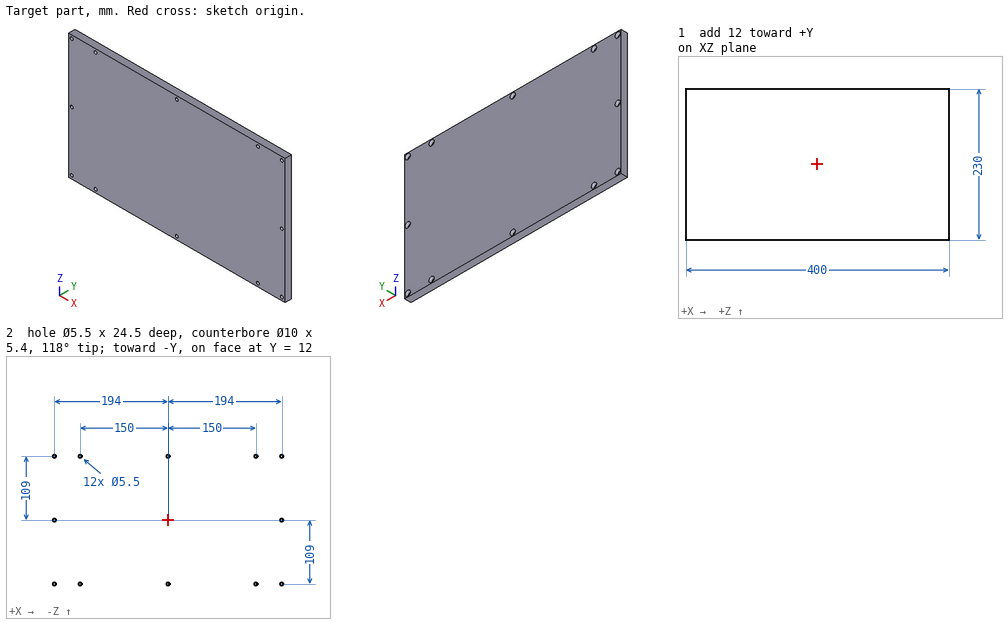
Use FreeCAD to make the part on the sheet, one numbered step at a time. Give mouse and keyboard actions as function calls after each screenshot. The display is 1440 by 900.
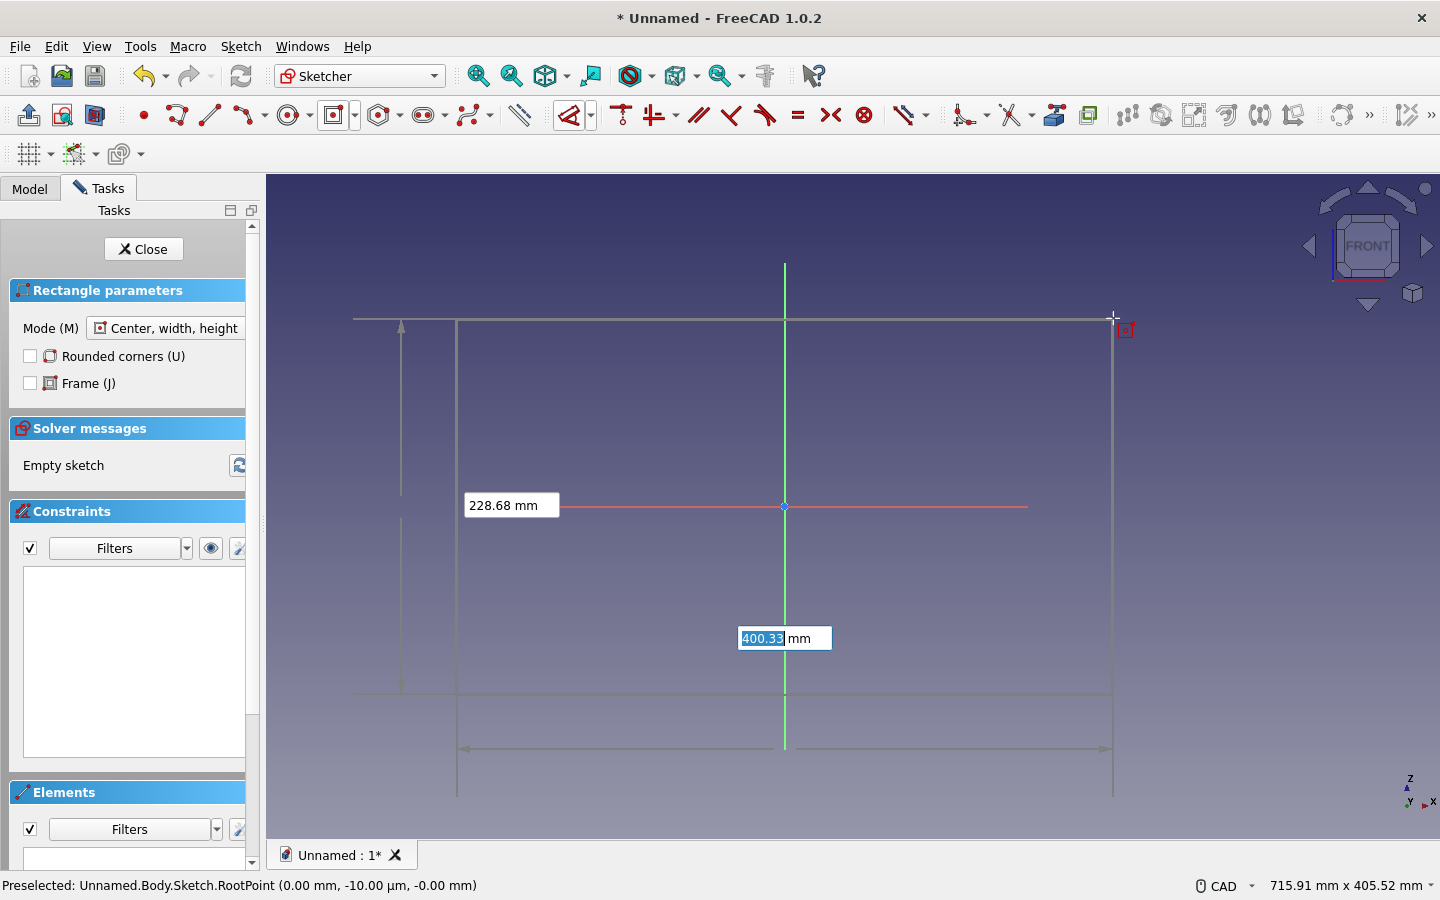
text(400)
key(Tab)
text(230)
key(Return)
key(Escape)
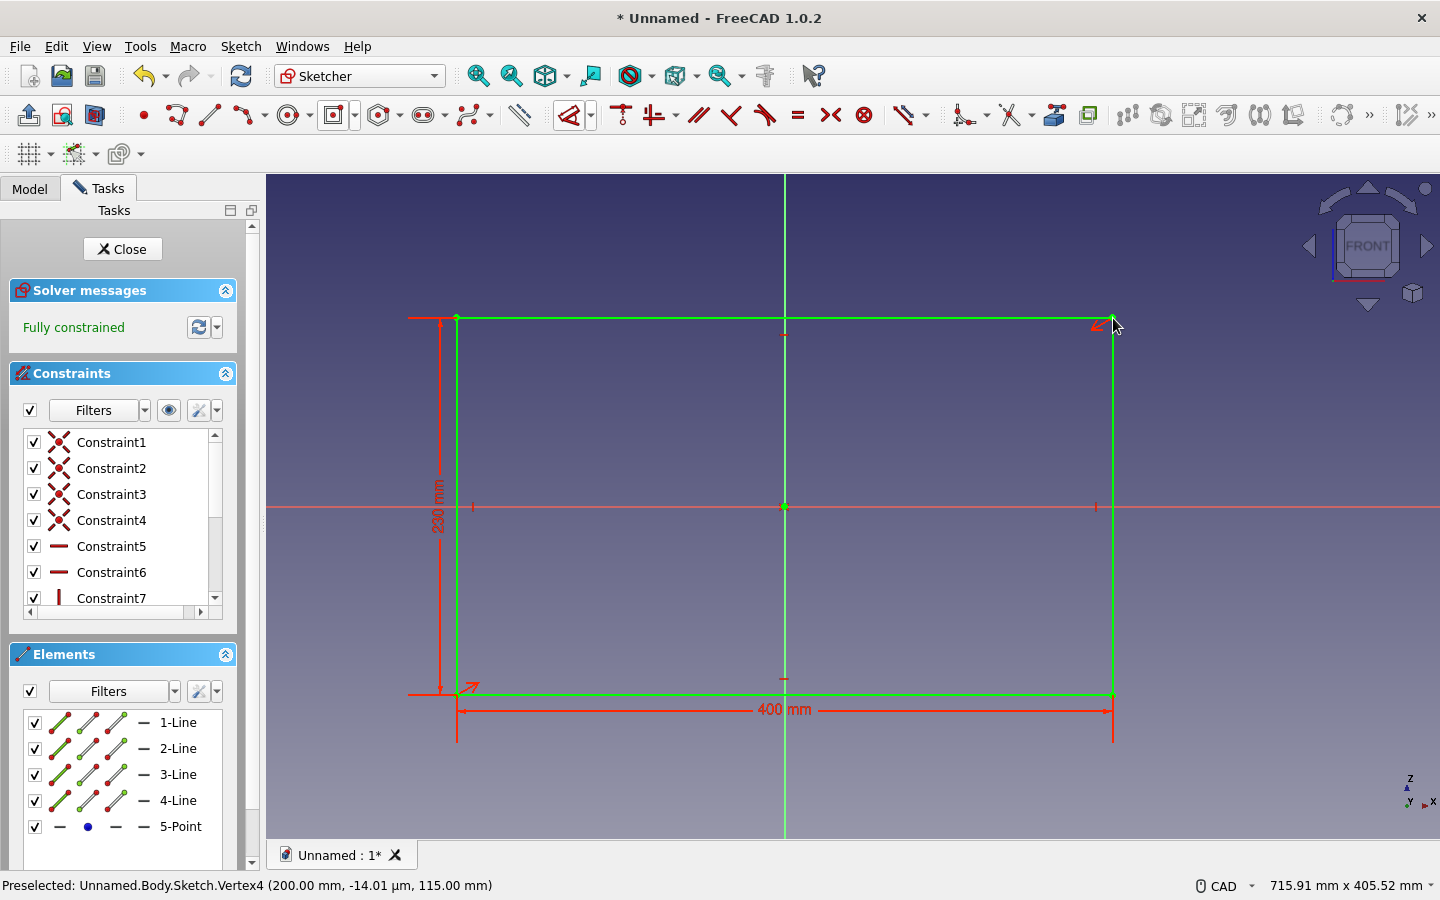
click(123, 249)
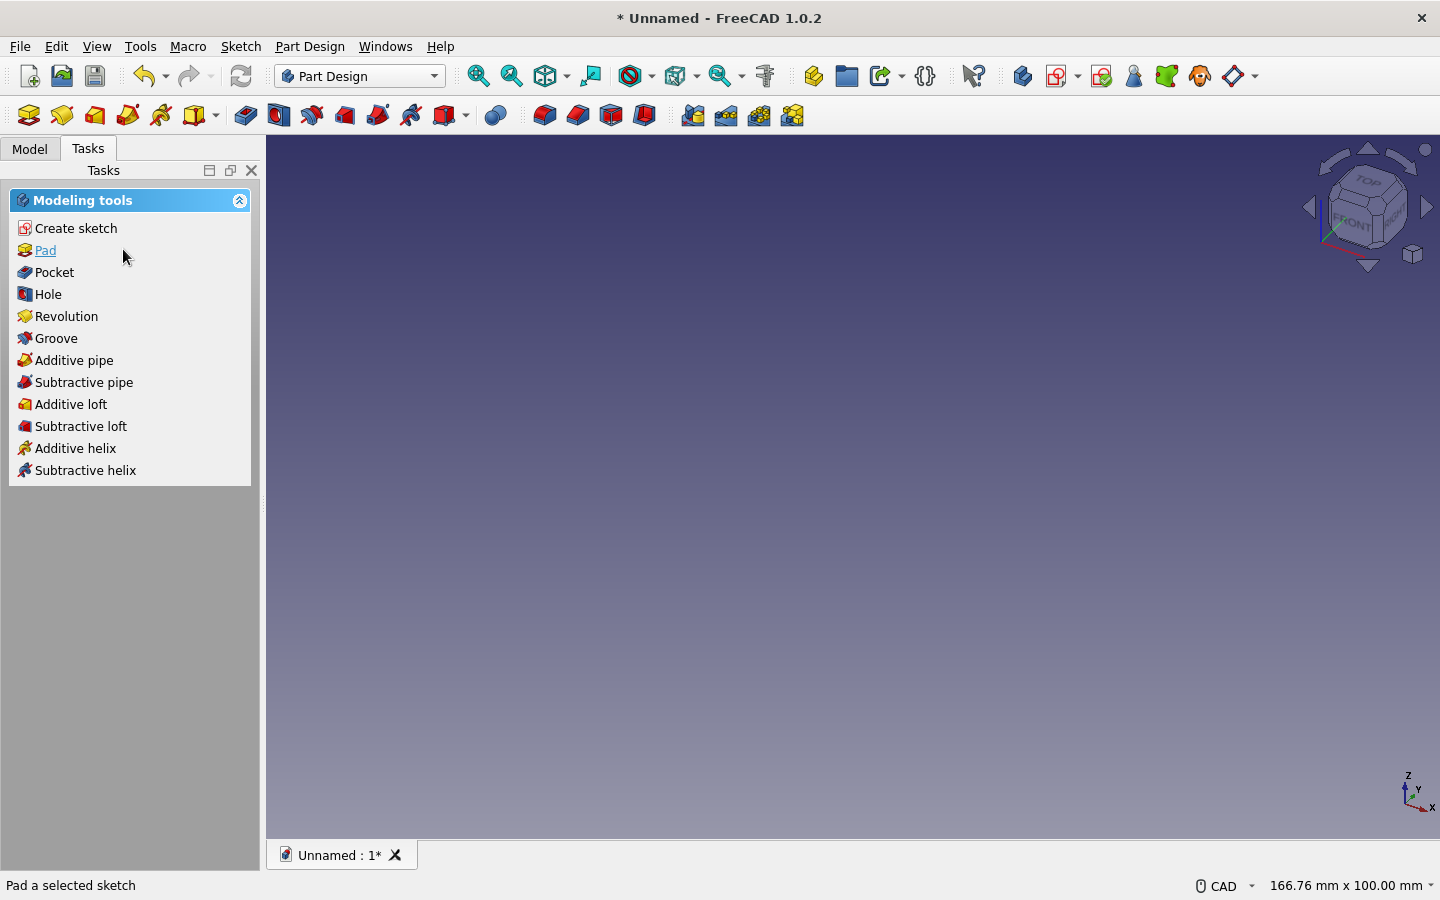
click(29, 116)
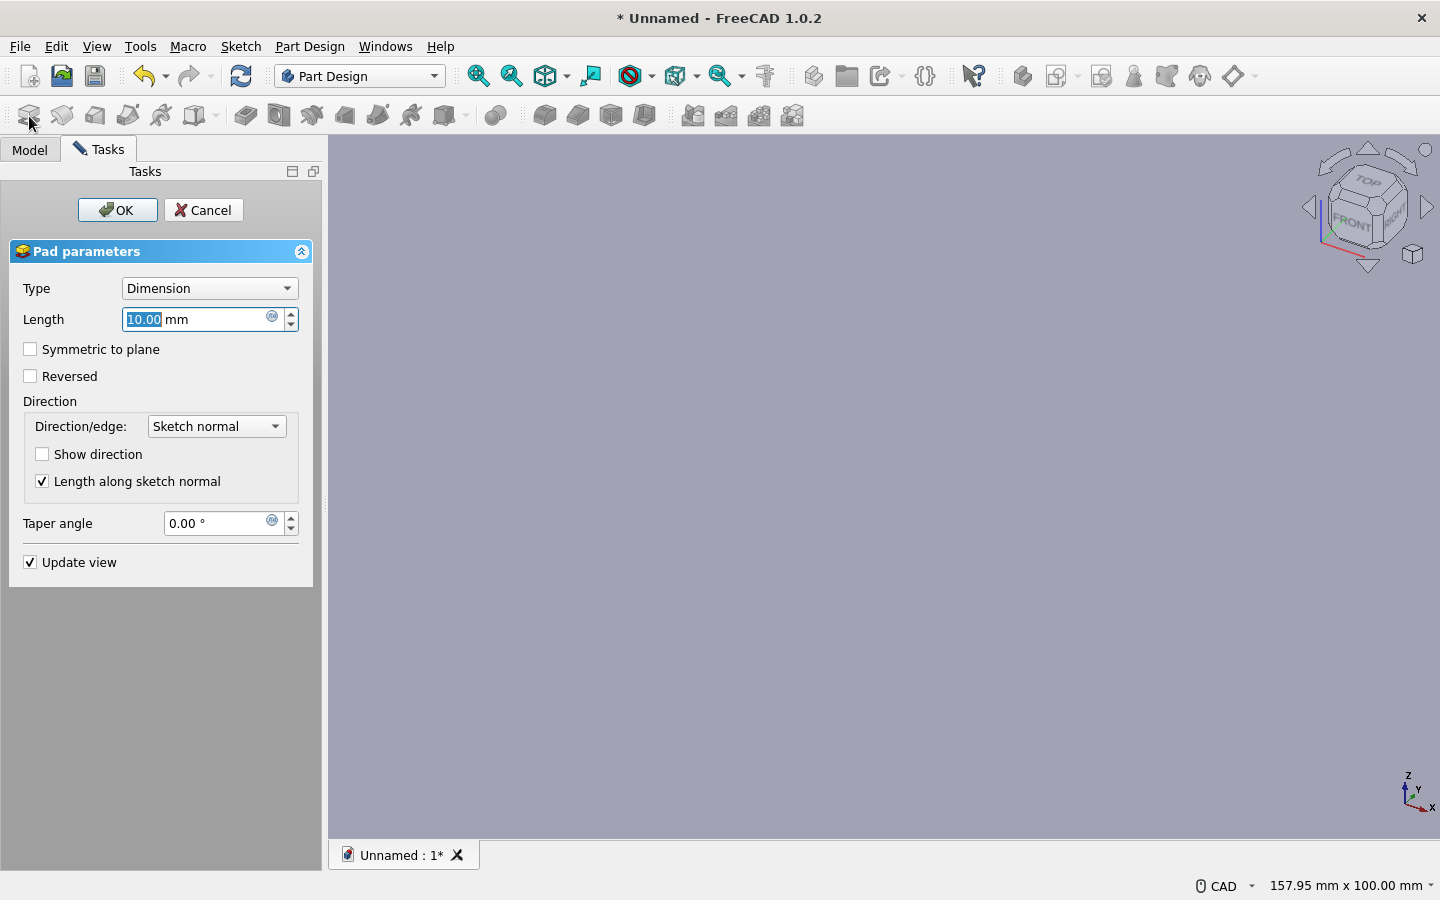
text(12)
key(Tab)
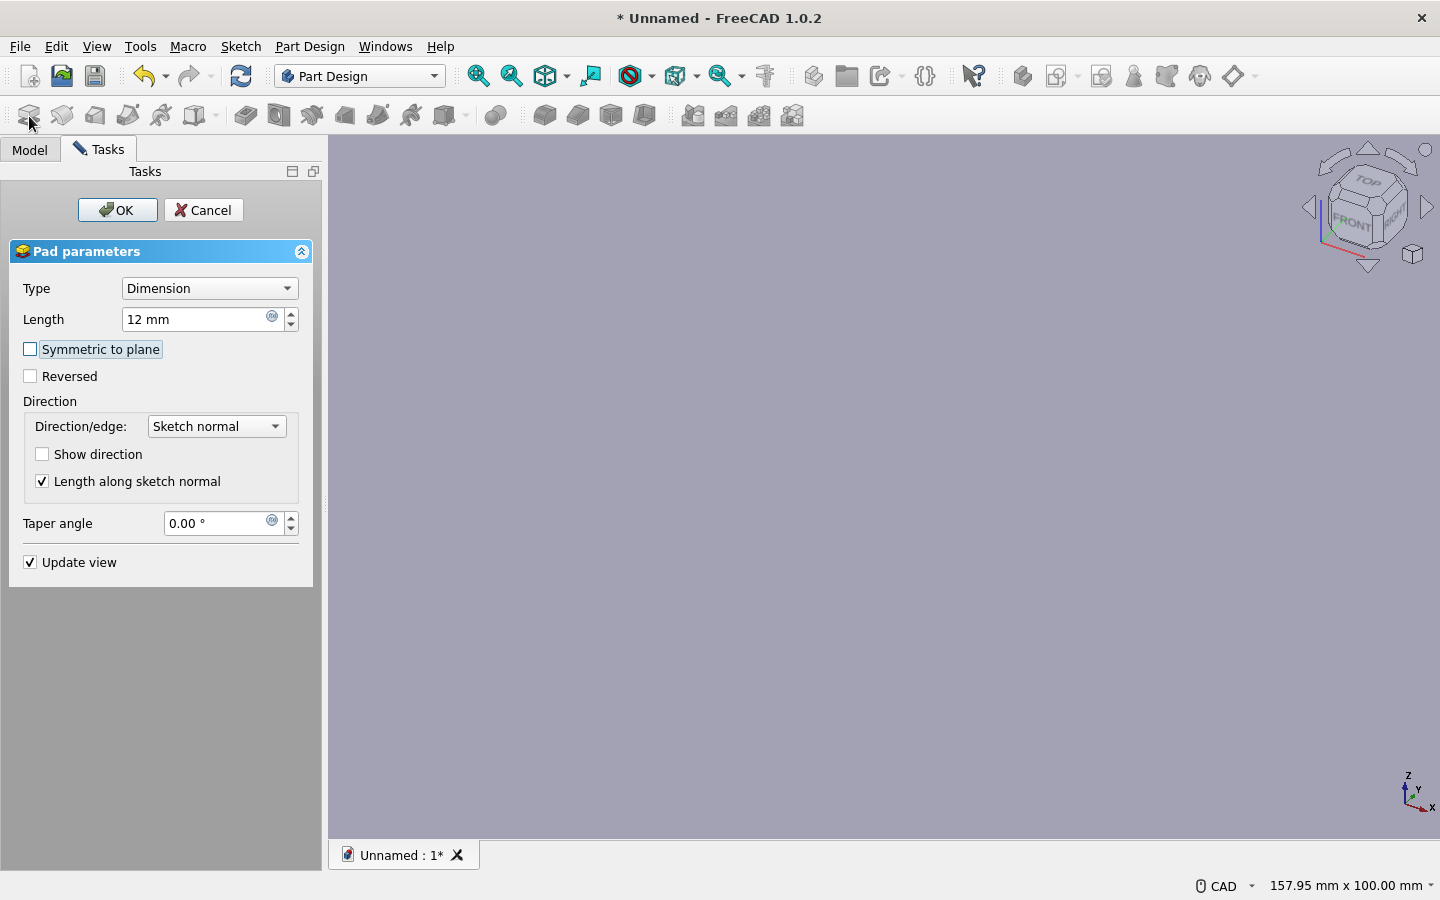
click(31, 376)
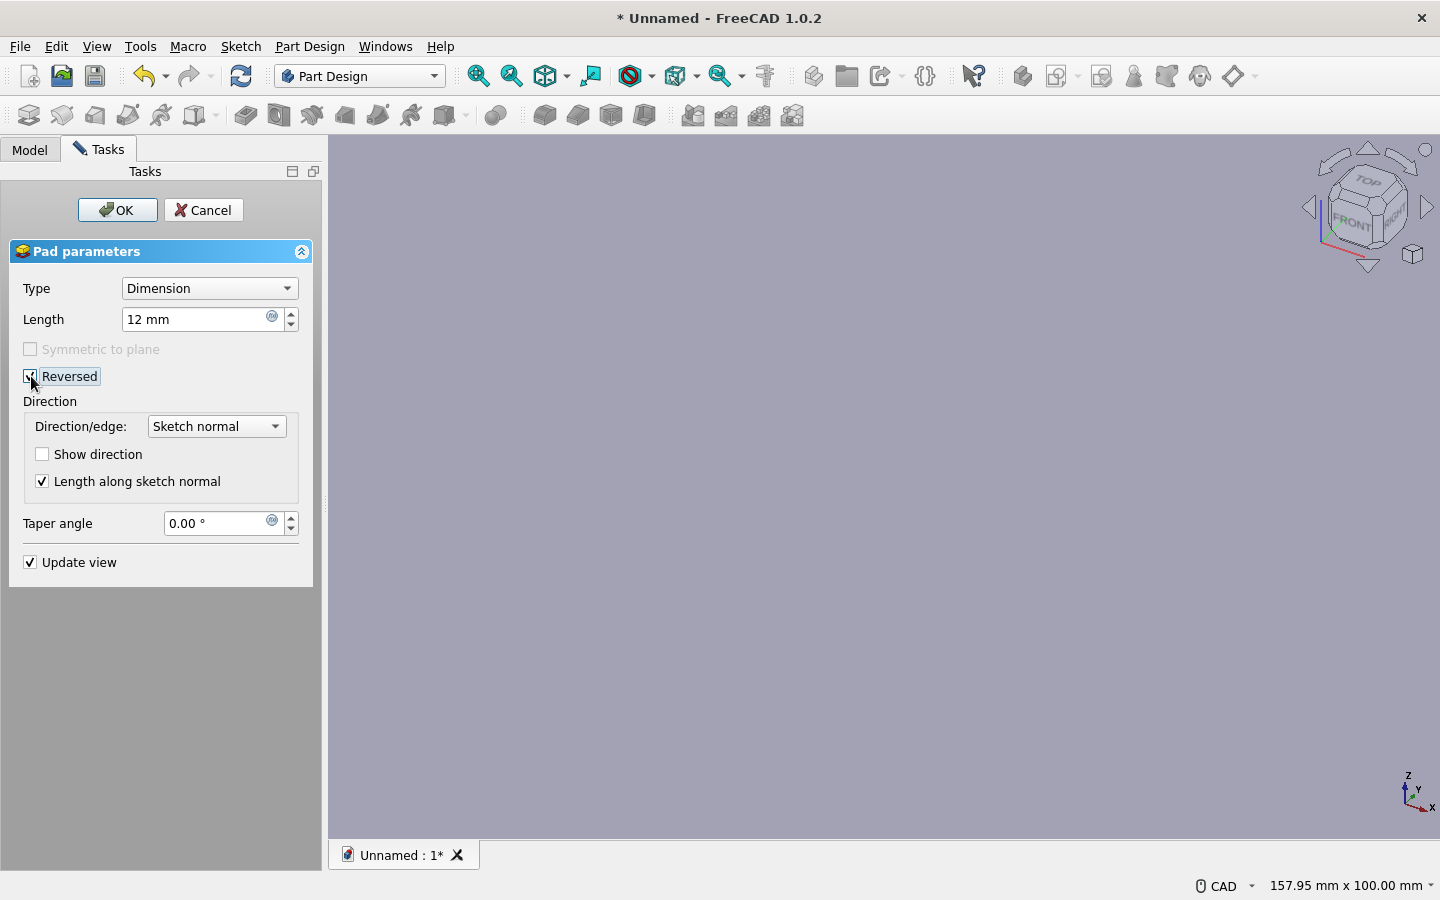
click(118, 210)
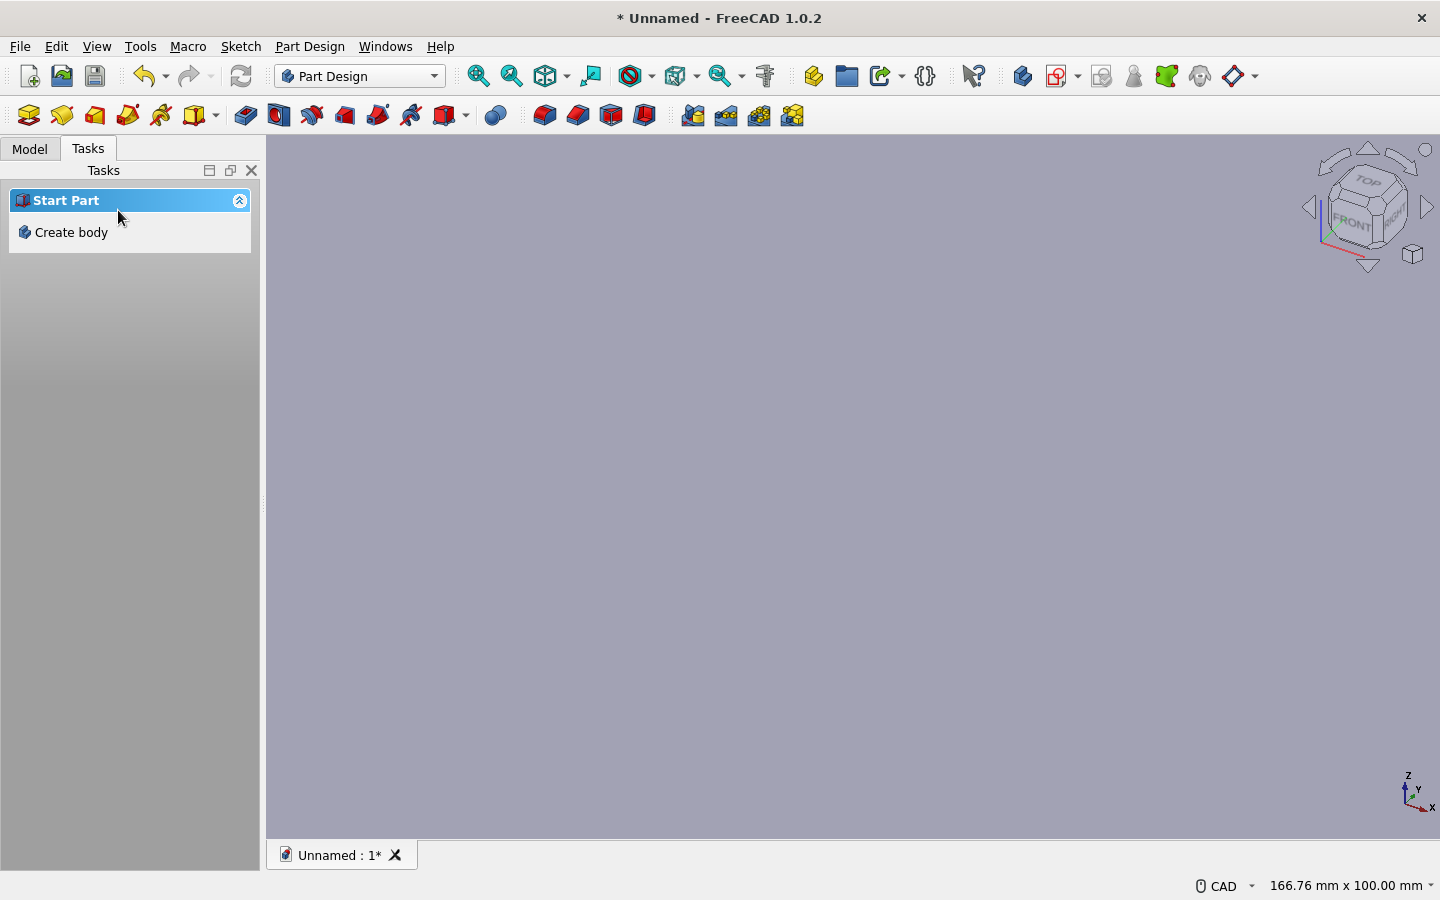
click(479, 76)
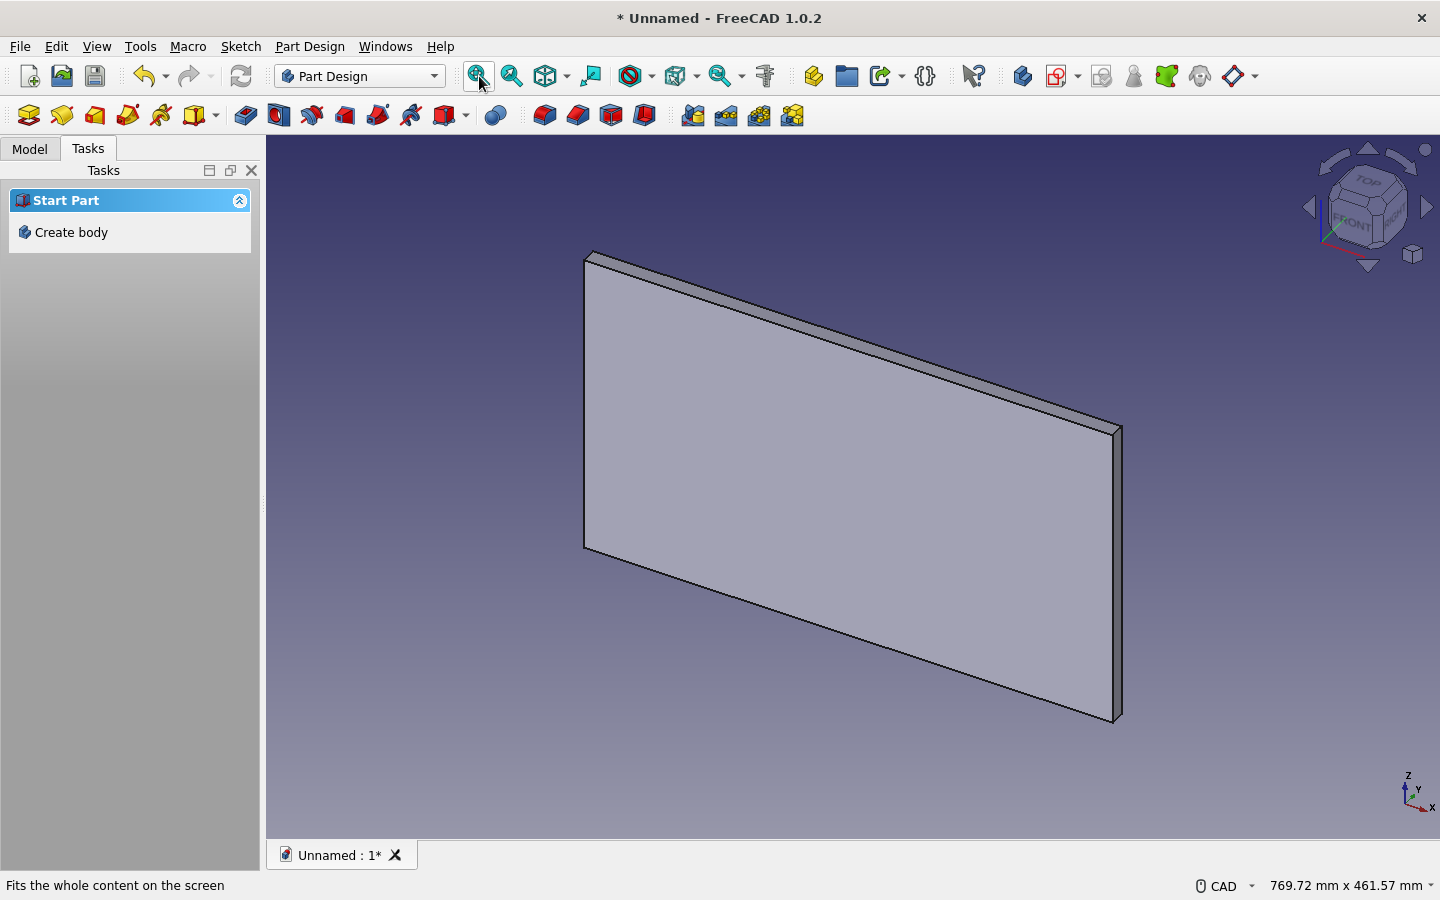
key(4)